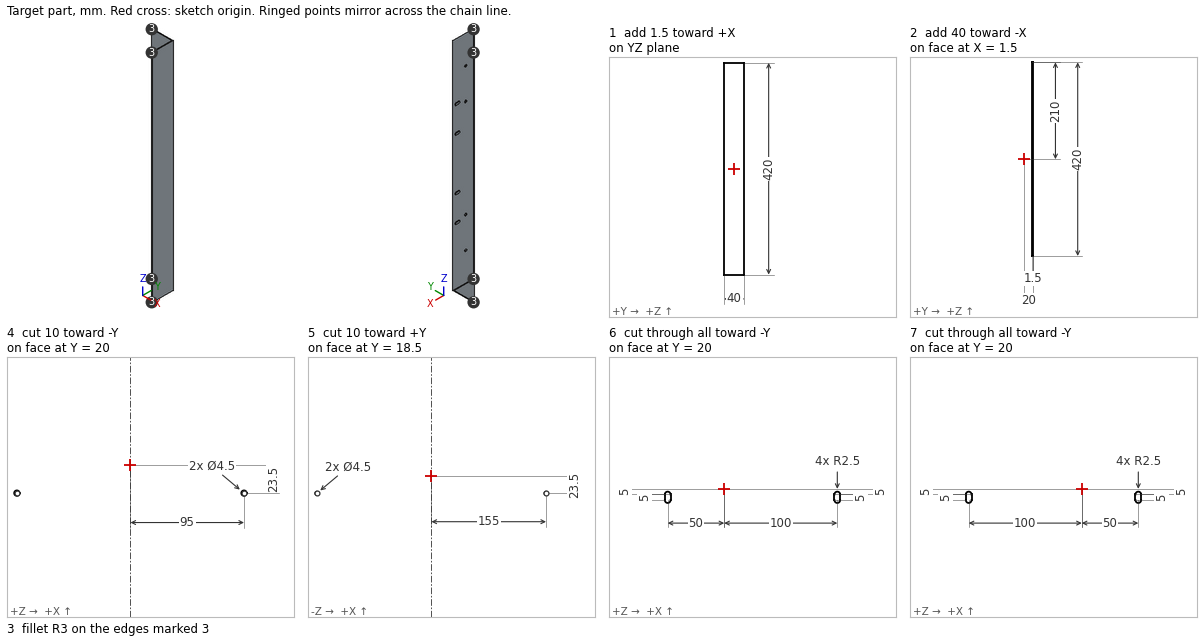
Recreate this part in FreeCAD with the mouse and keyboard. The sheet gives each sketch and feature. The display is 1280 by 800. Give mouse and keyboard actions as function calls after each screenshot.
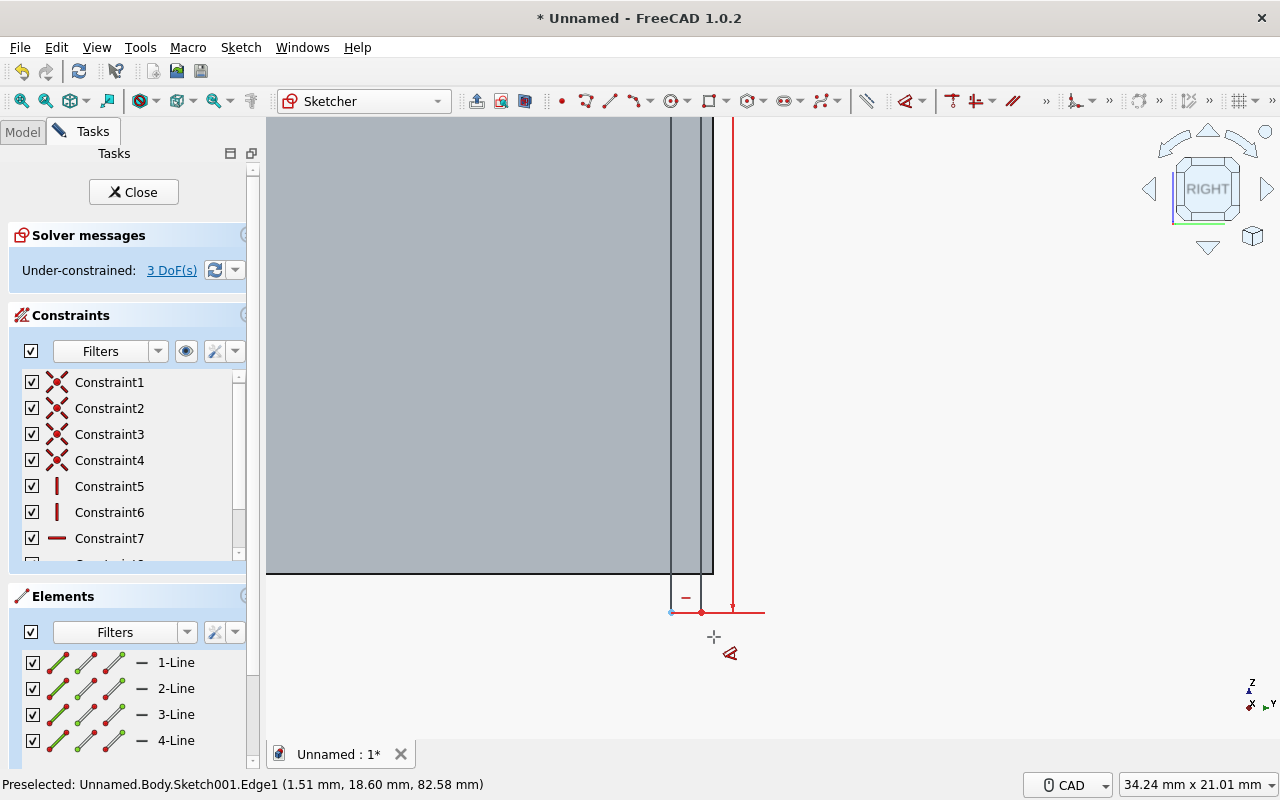
click(686, 613)
click(686, 647)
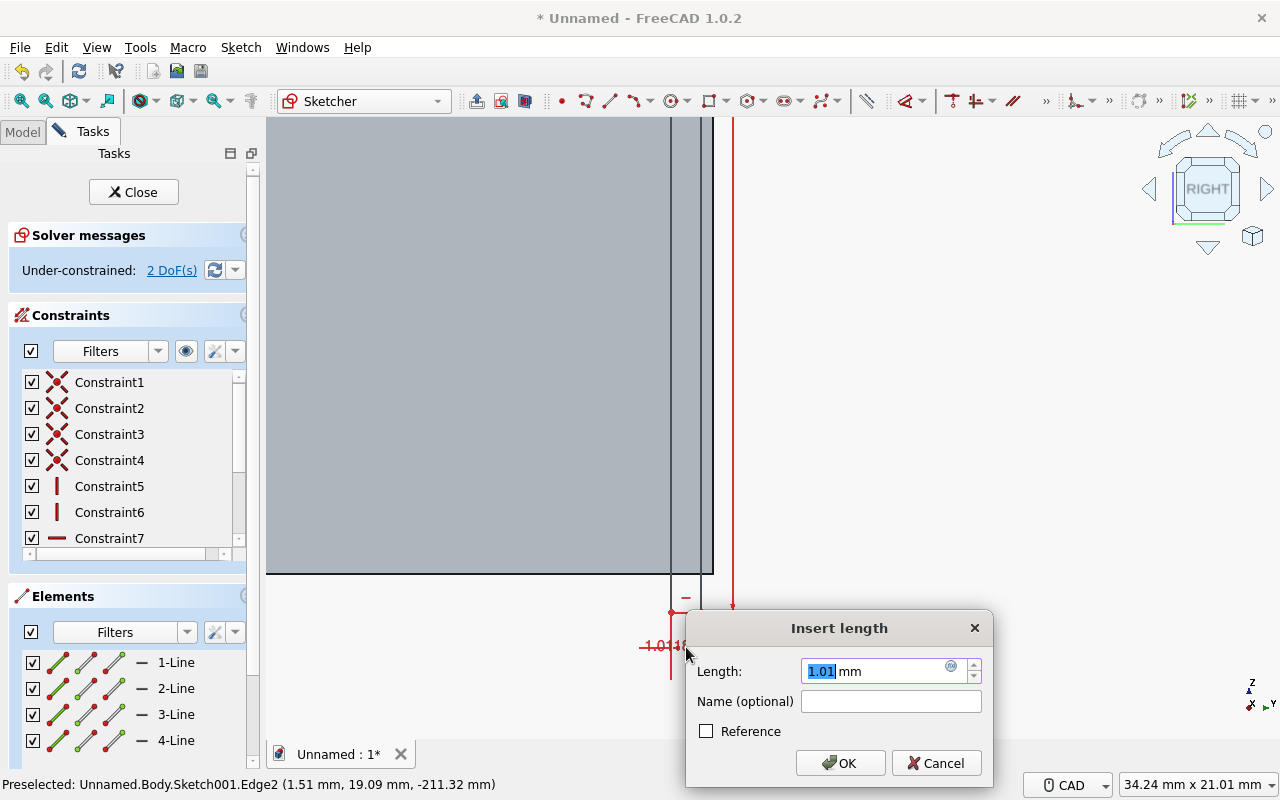
text(1.5)
key(Return)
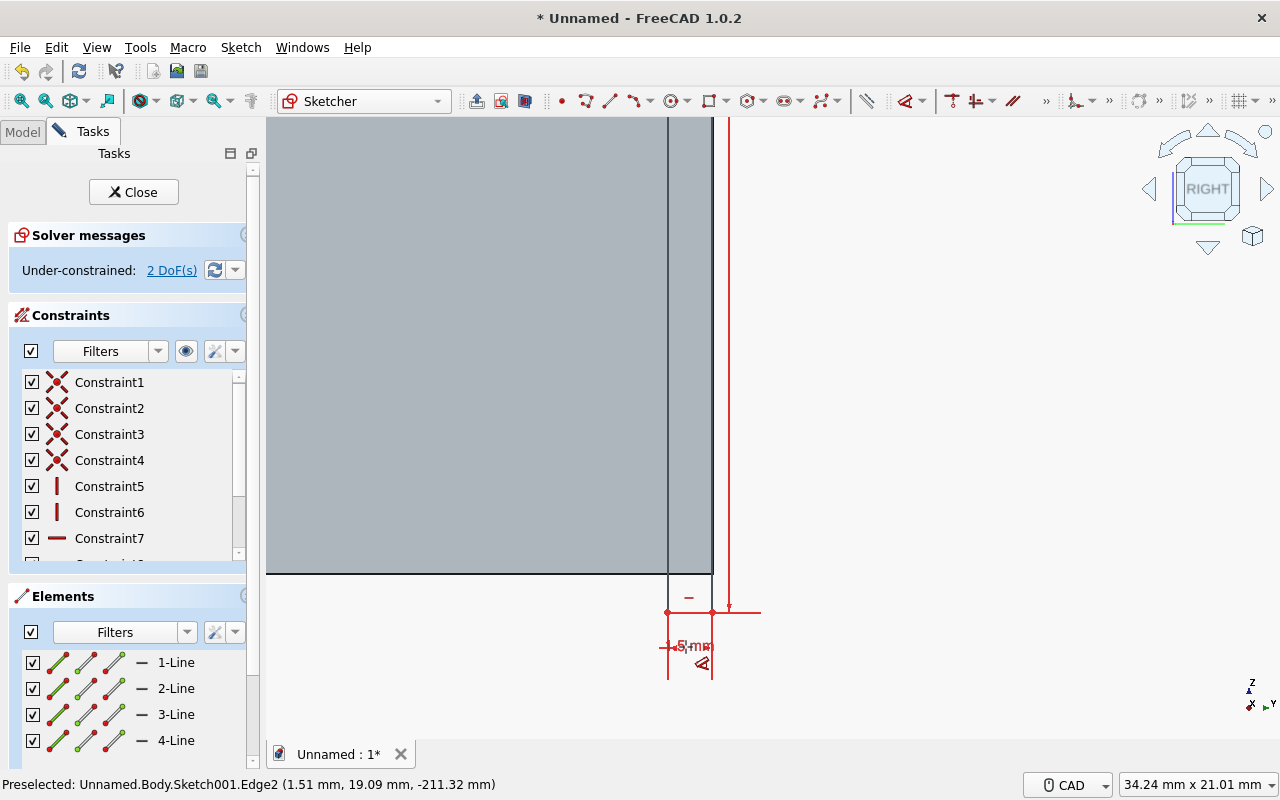
scroll(717, 686, down, 16)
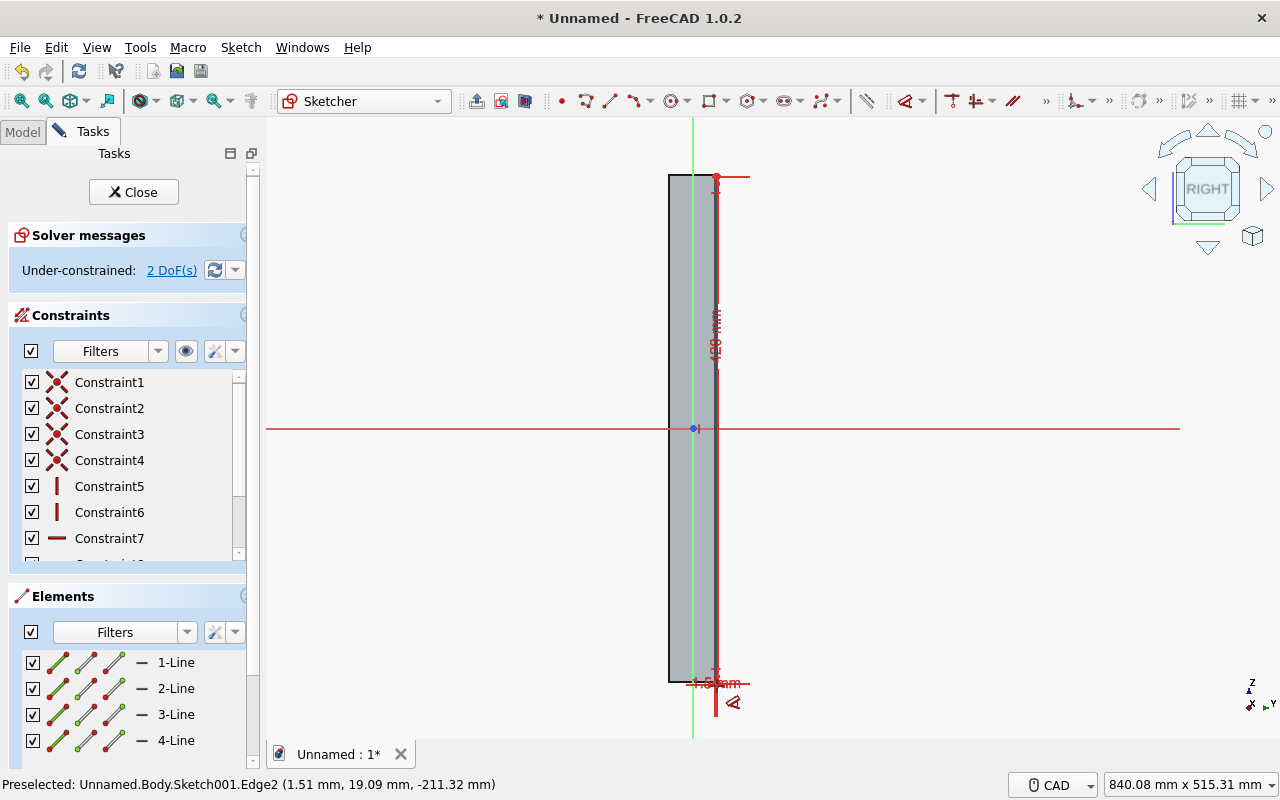
scroll(717, 684, up, 10)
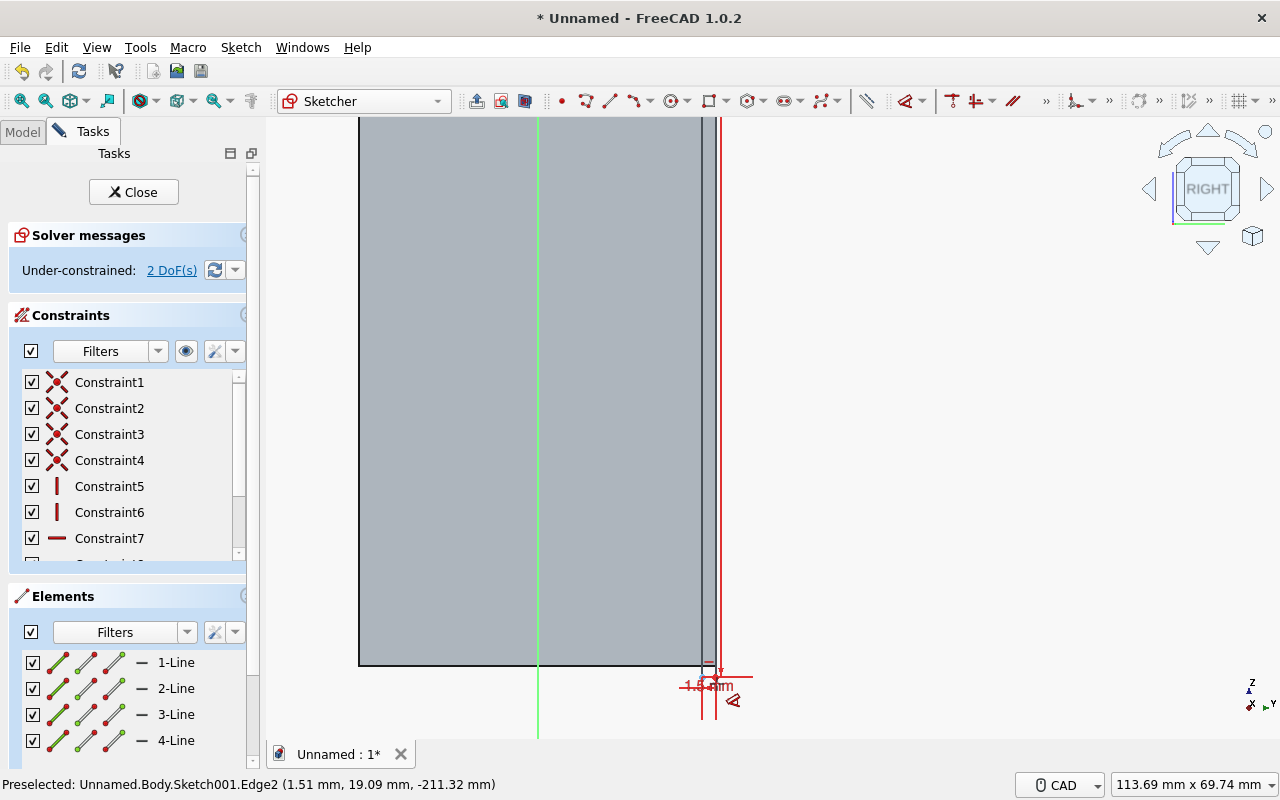
click(716, 677)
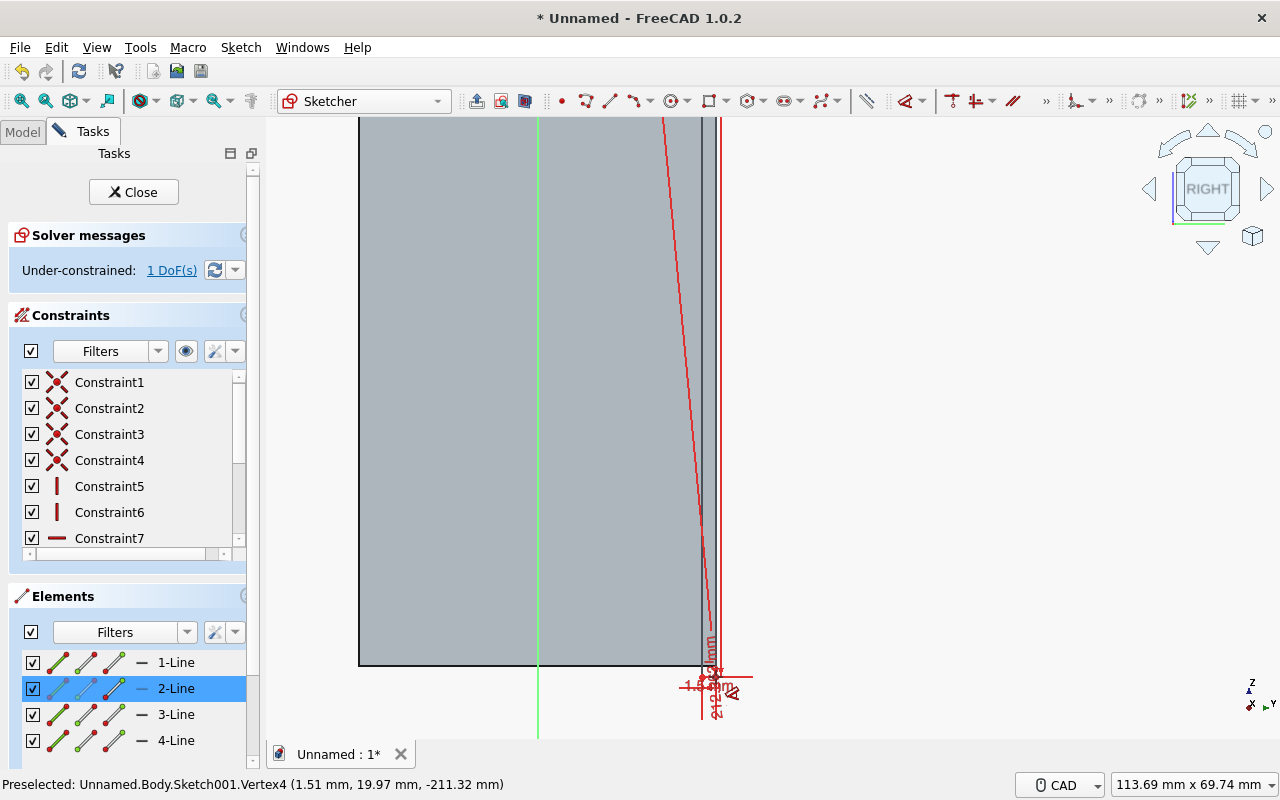
key(Escape)
key(Escape)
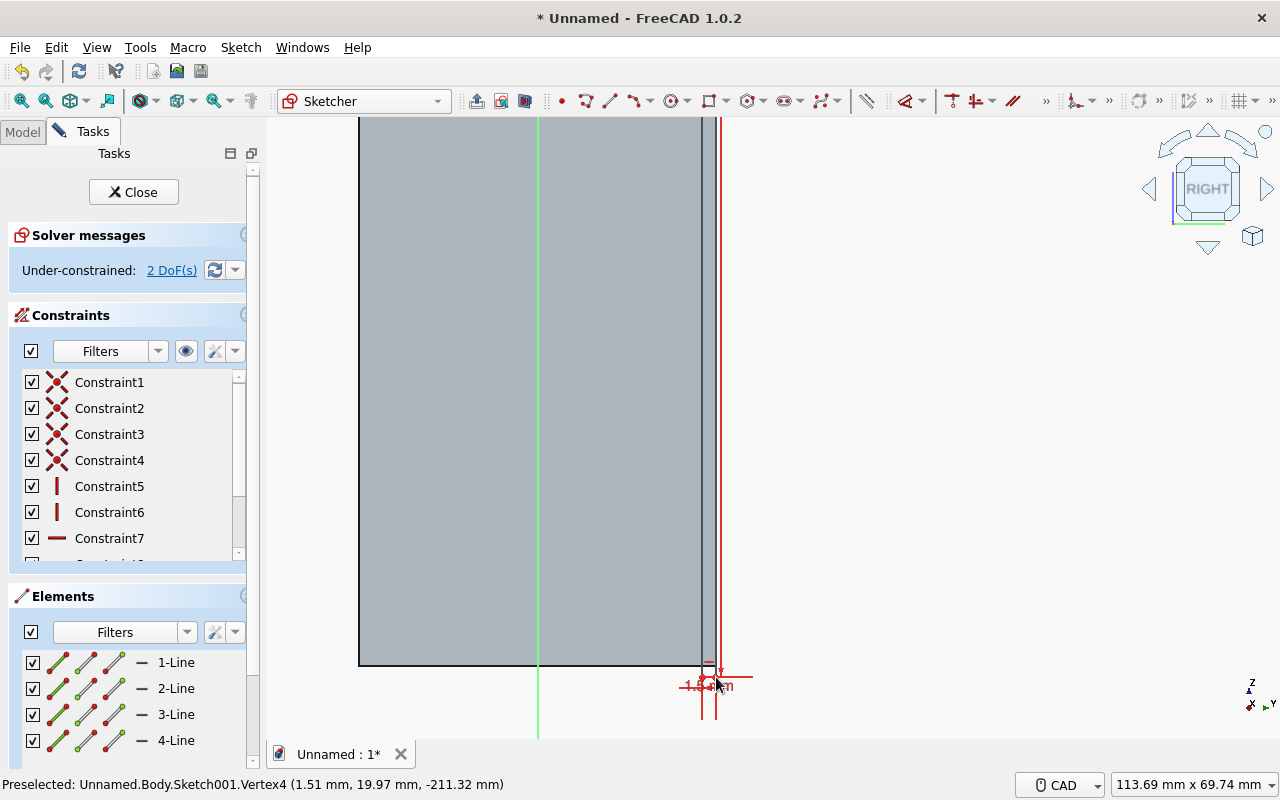
click(716, 677)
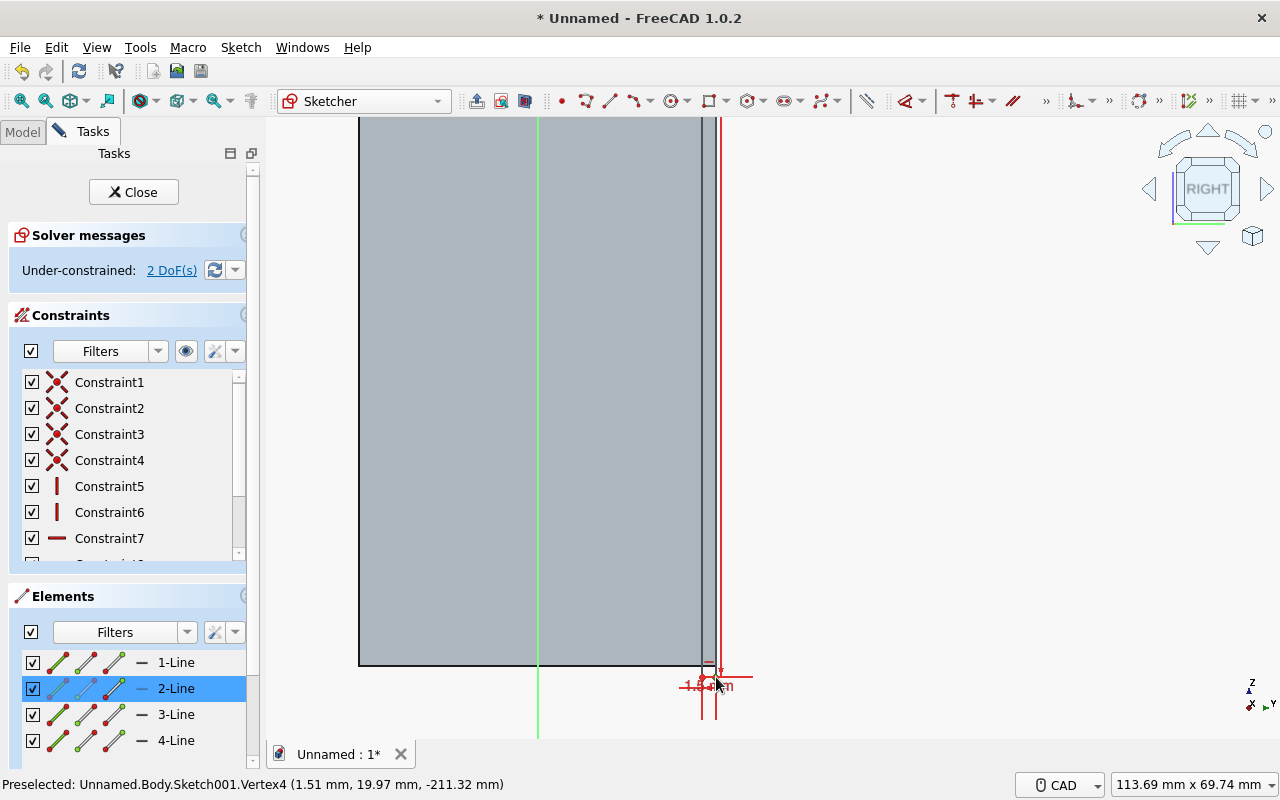
key(l)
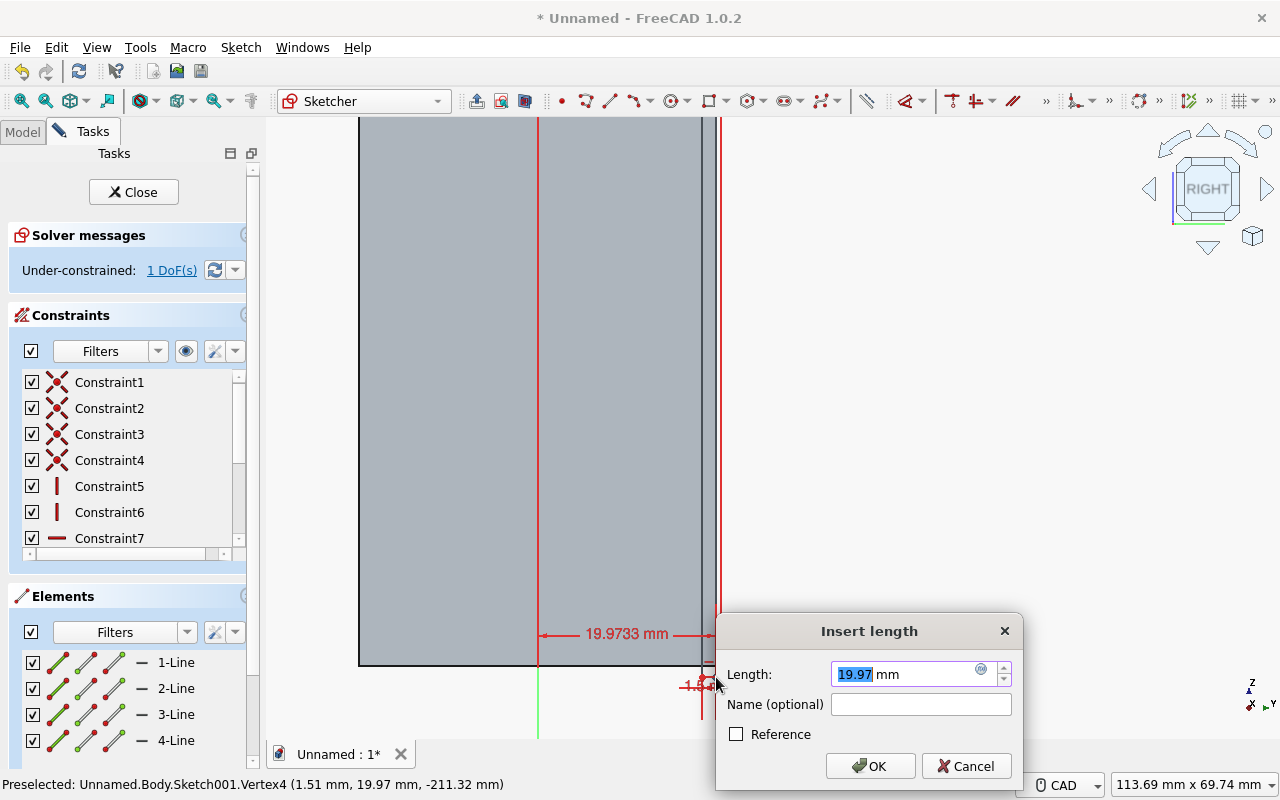
text(20)
key(Return)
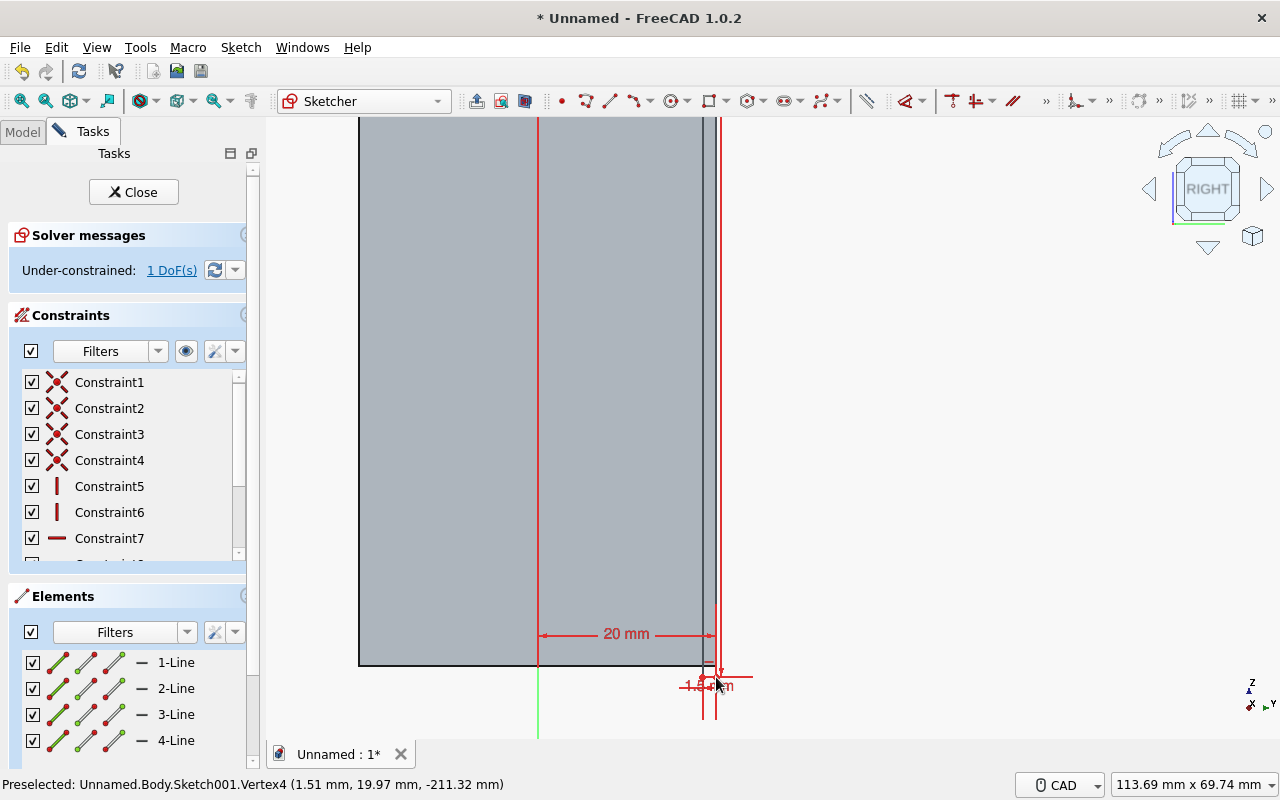
scroll(714, 632, down, 11)